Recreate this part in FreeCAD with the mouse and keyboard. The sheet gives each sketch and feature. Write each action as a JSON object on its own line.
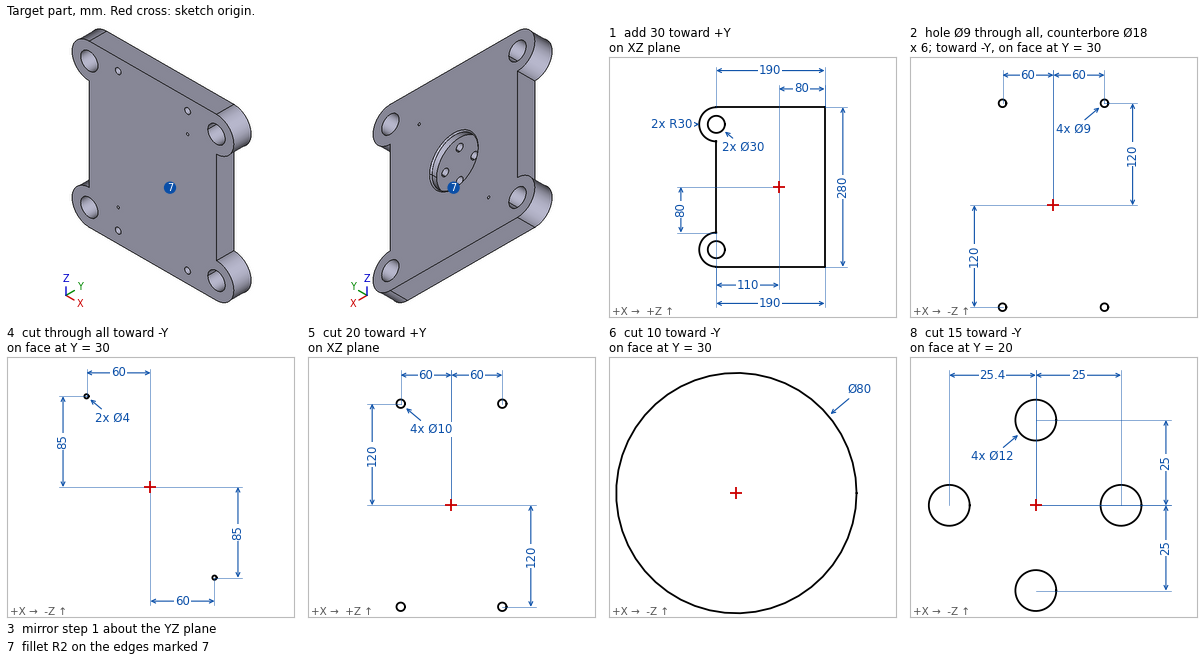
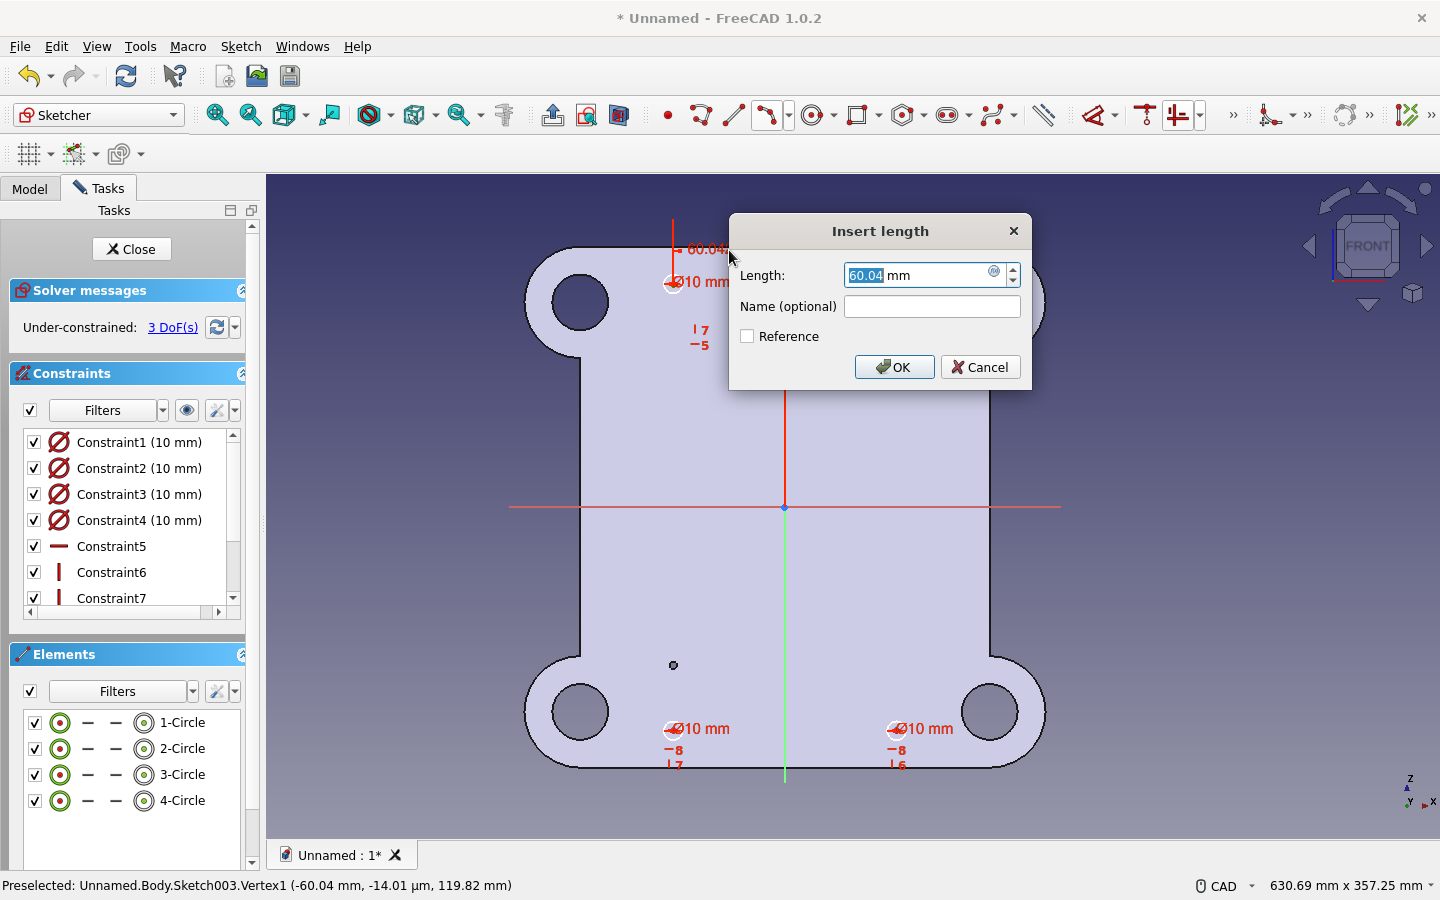
{"action": "type", "text": "60"}
{"action": "key", "text": "Return"}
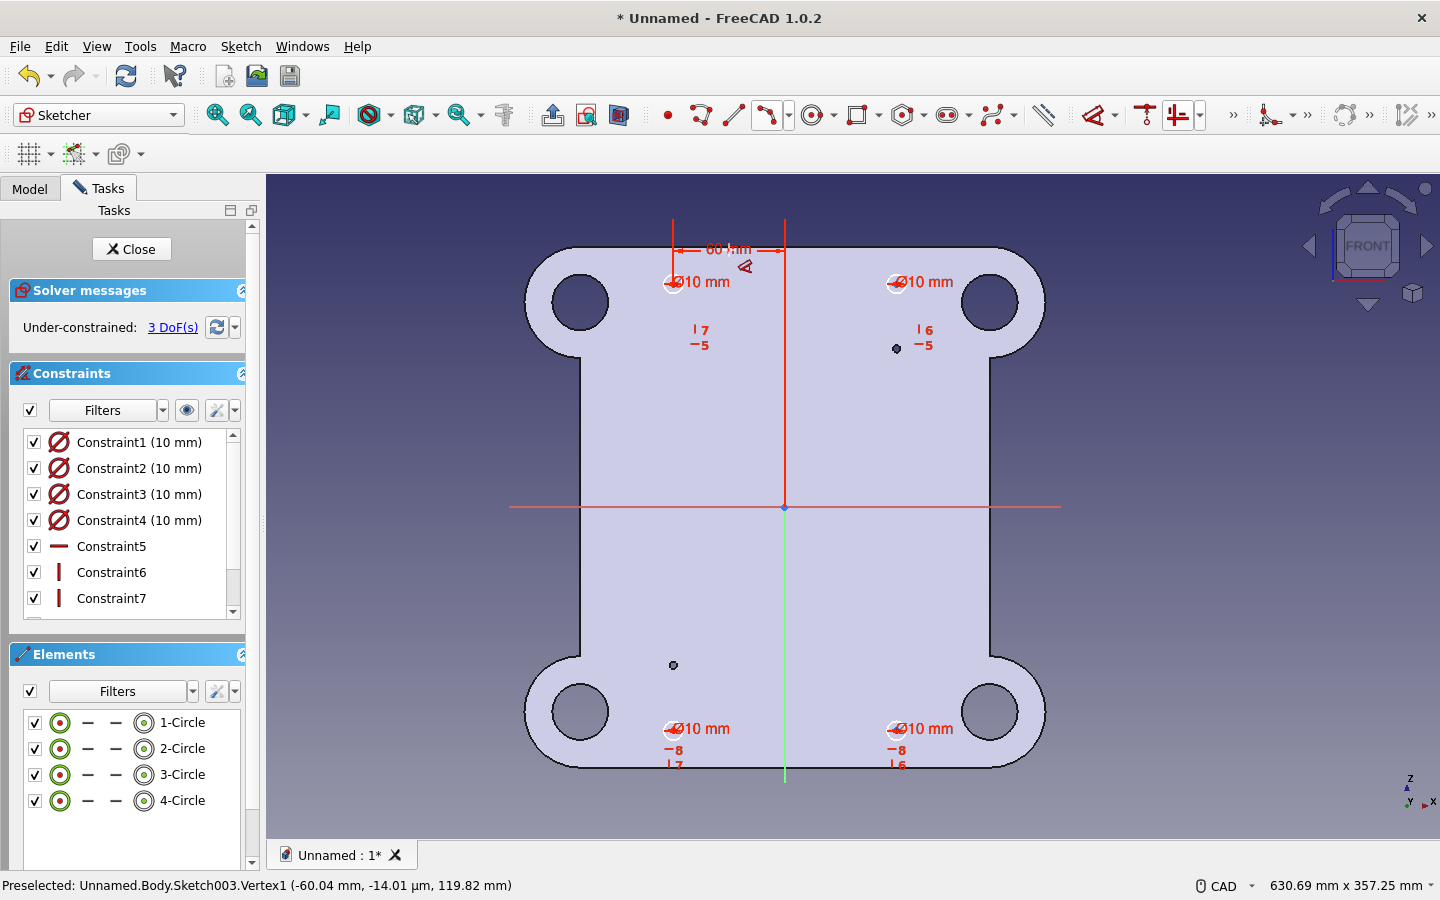
{"action": "left_click", "coordinate": [897, 284]}
{"action": "left_click", "coordinate": [841, 250]}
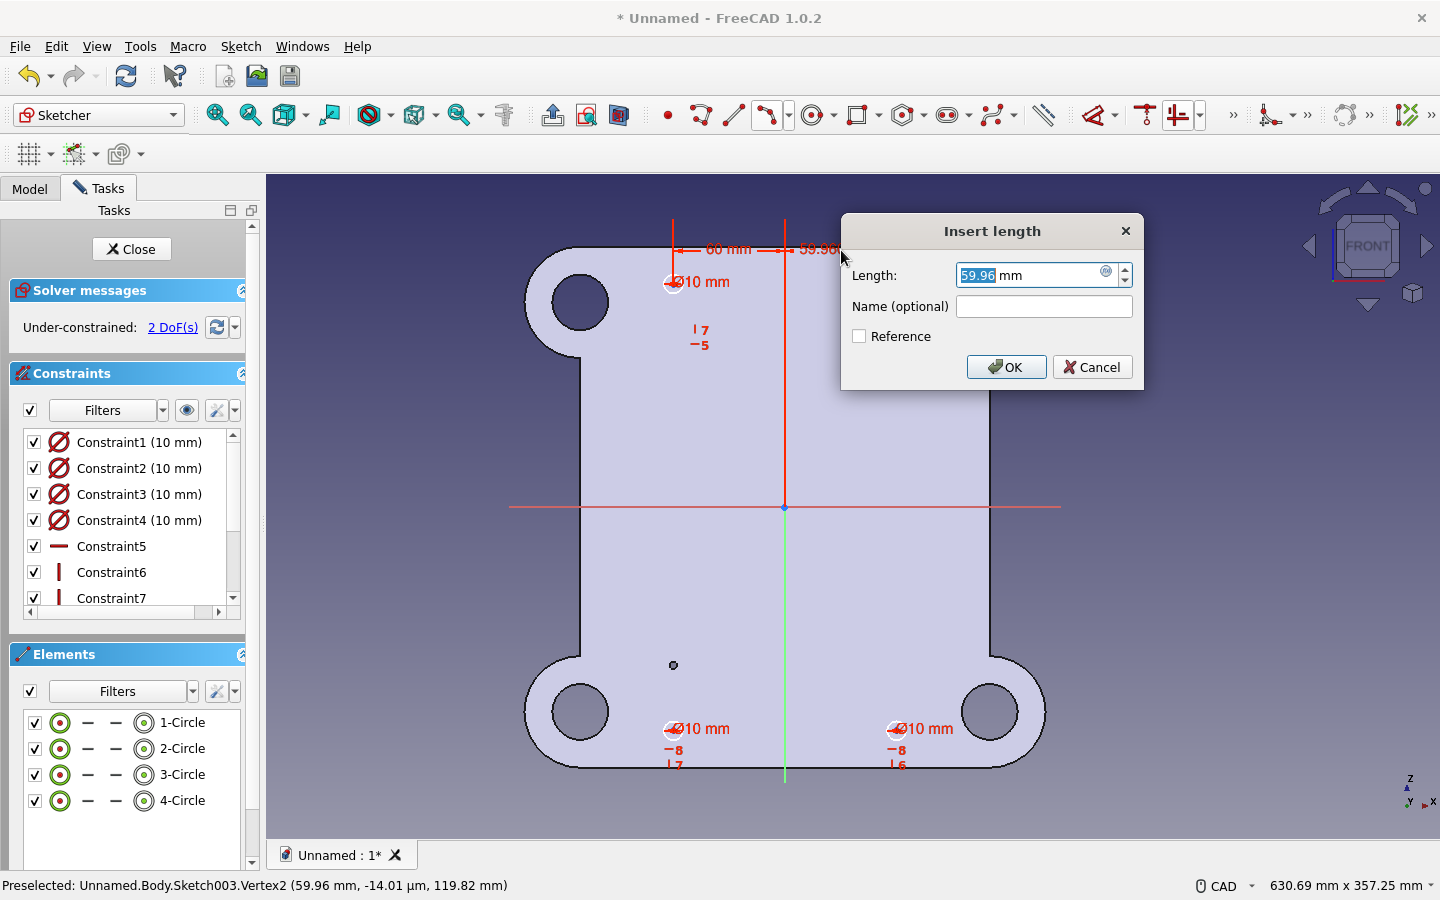
{"action": "type", "text": "60"}
{"action": "key", "text": "Return"}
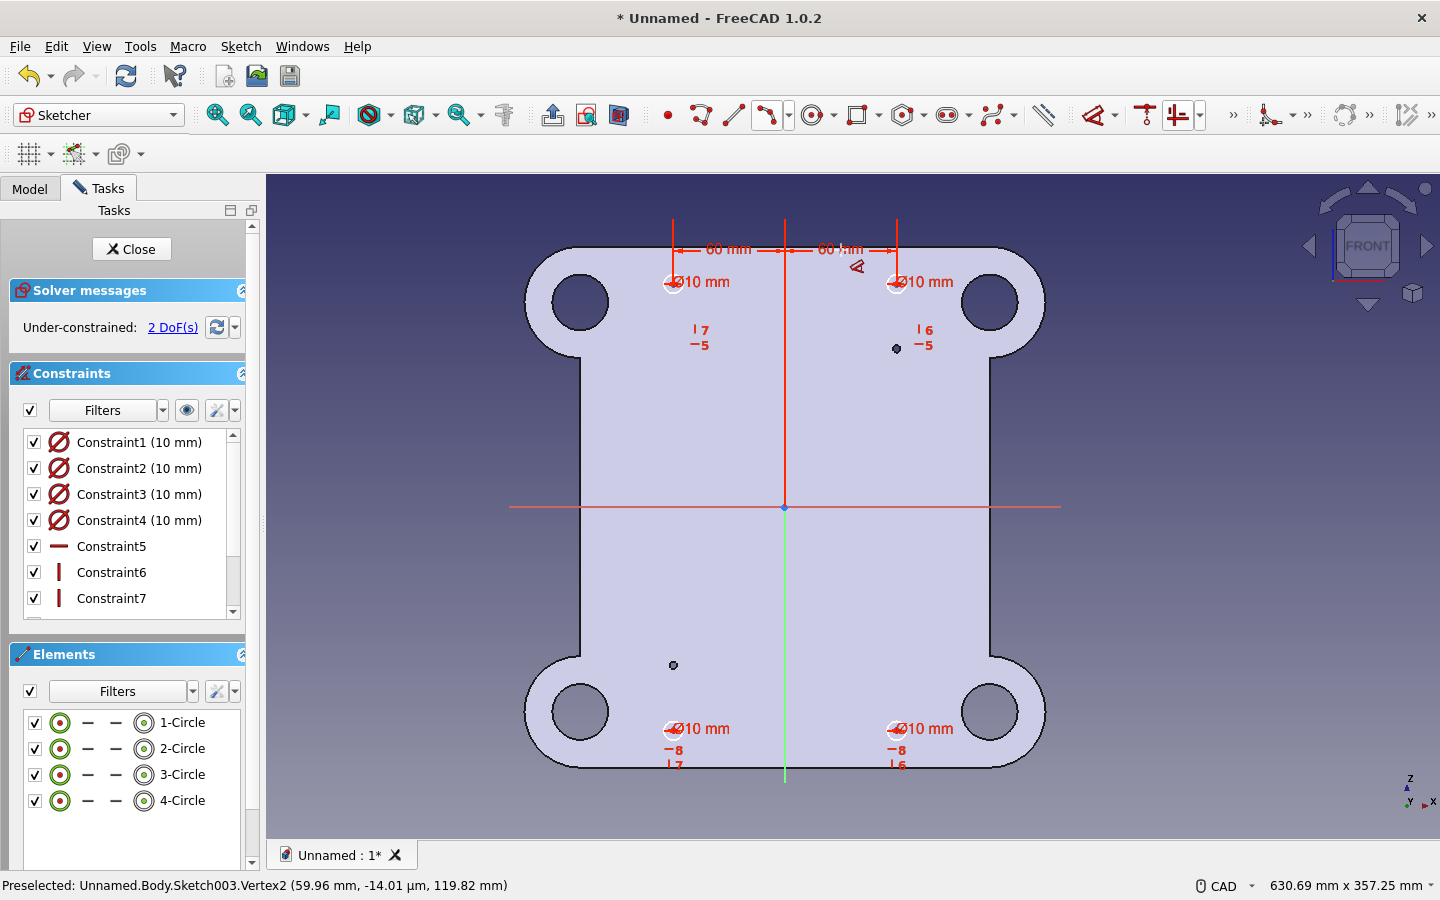
{"action": "left_click", "coordinate": [673, 284]}
{"action": "left_click", "coordinate": [639, 396]}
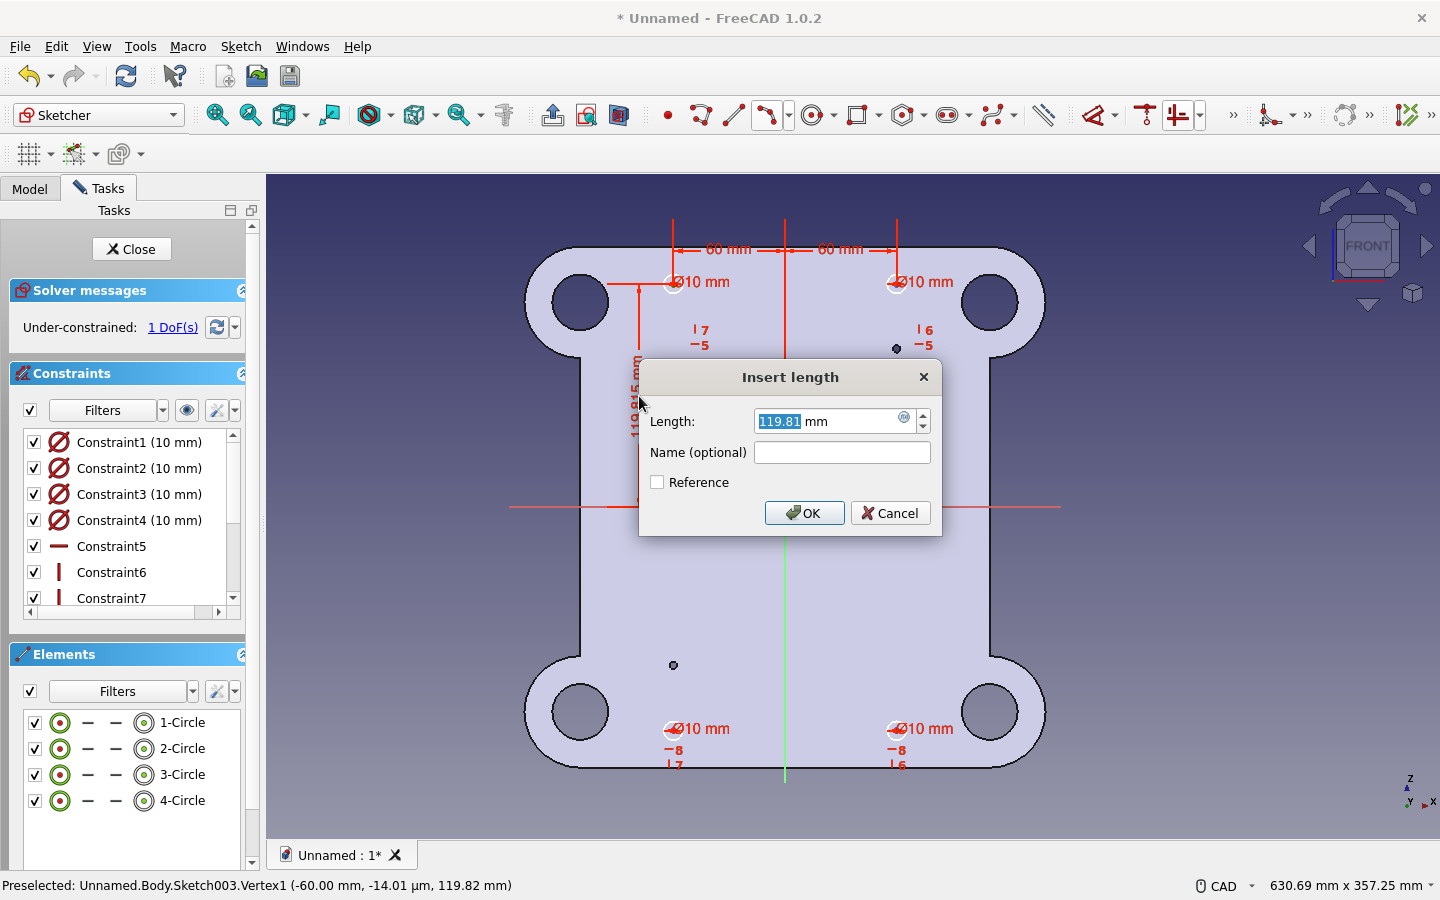
{"action": "type", "text": "120"}
{"action": "key", "text": "Return"}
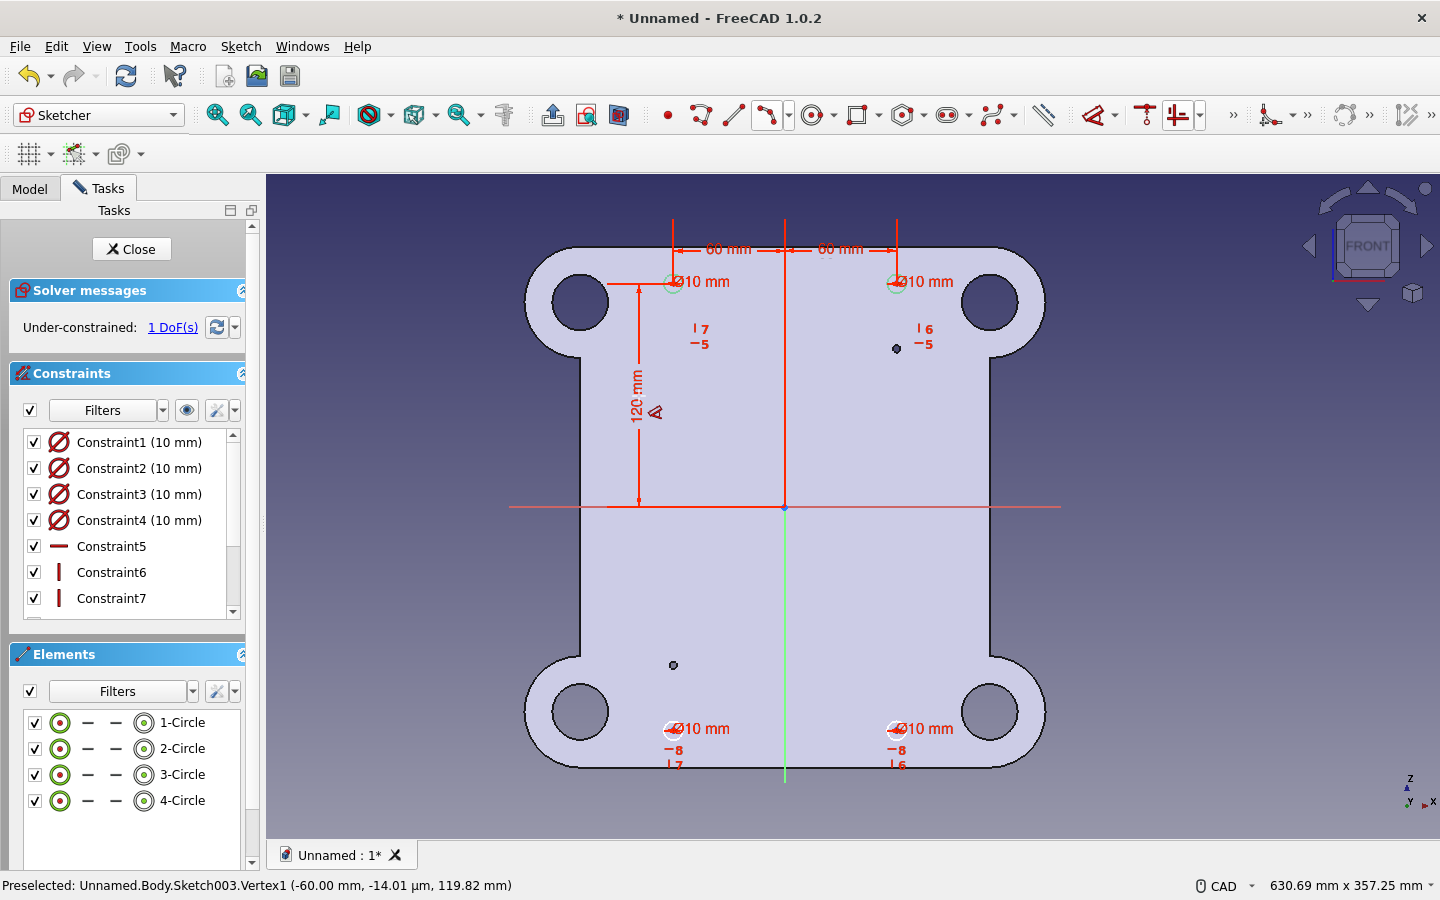
{"action": "left_click", "coordinate": [897, 731]}
{"action": "left_click", "coordinate": [931, 619]}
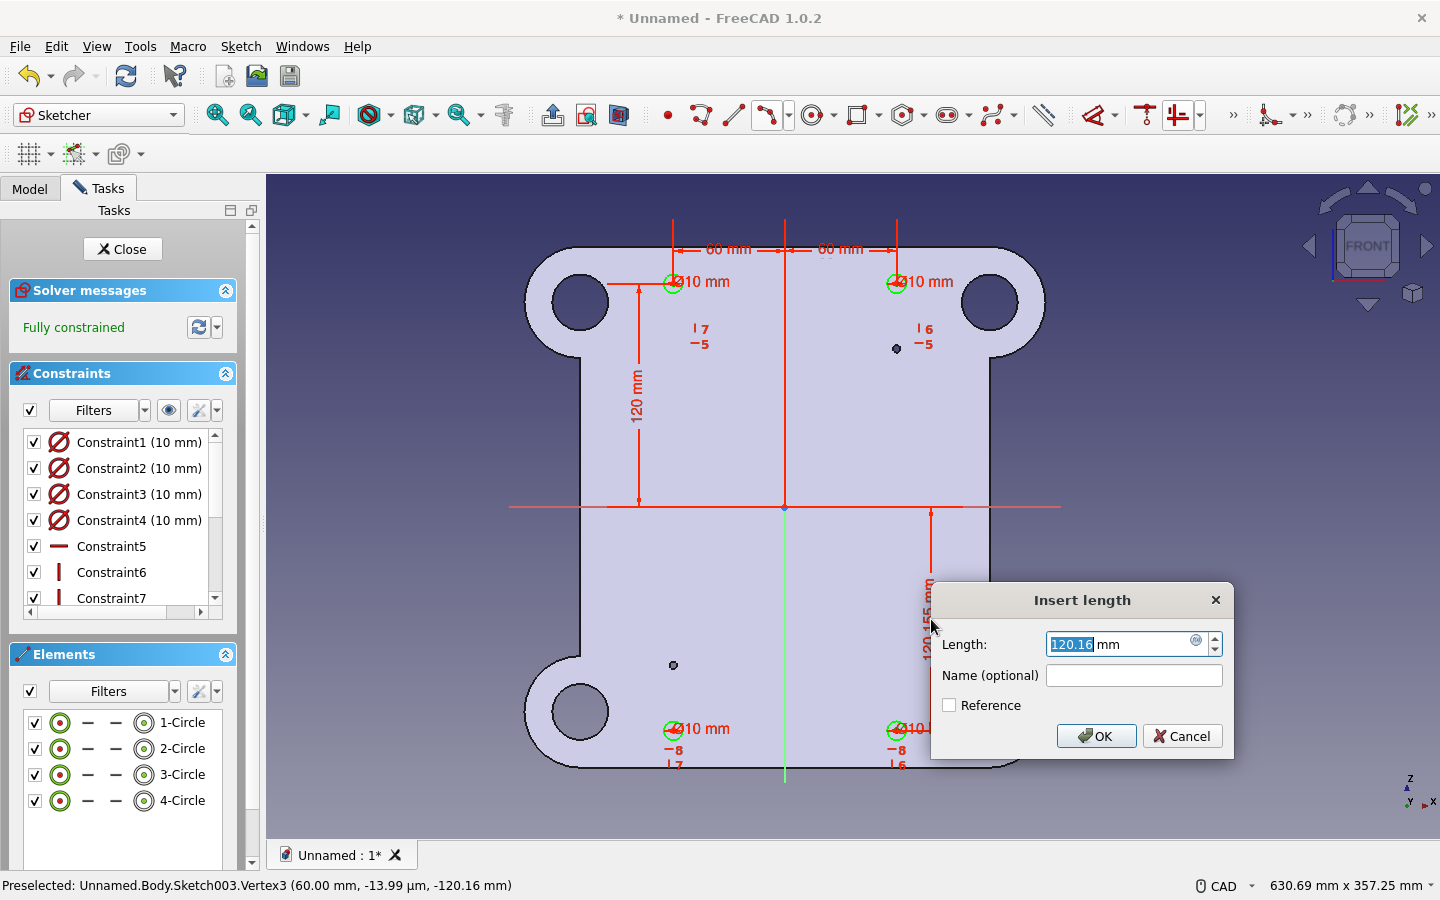
{"action": "type", "text": "120"}
{"action": "key", "text": "Return"}
{"action": "key", "text": "Escape"}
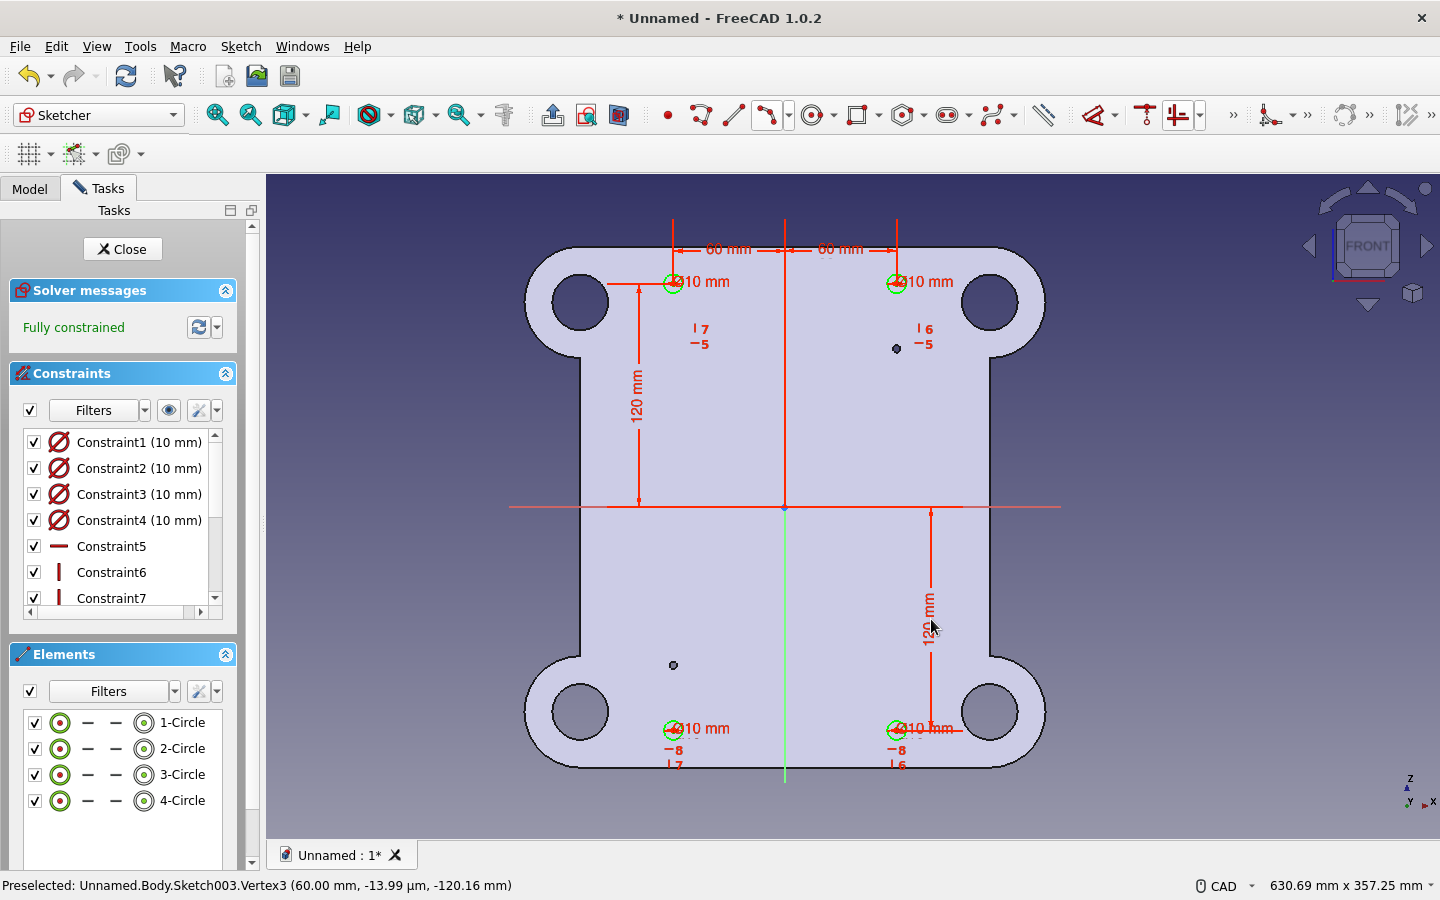
{"action": "left_click", "coordinate": [123, 249]}